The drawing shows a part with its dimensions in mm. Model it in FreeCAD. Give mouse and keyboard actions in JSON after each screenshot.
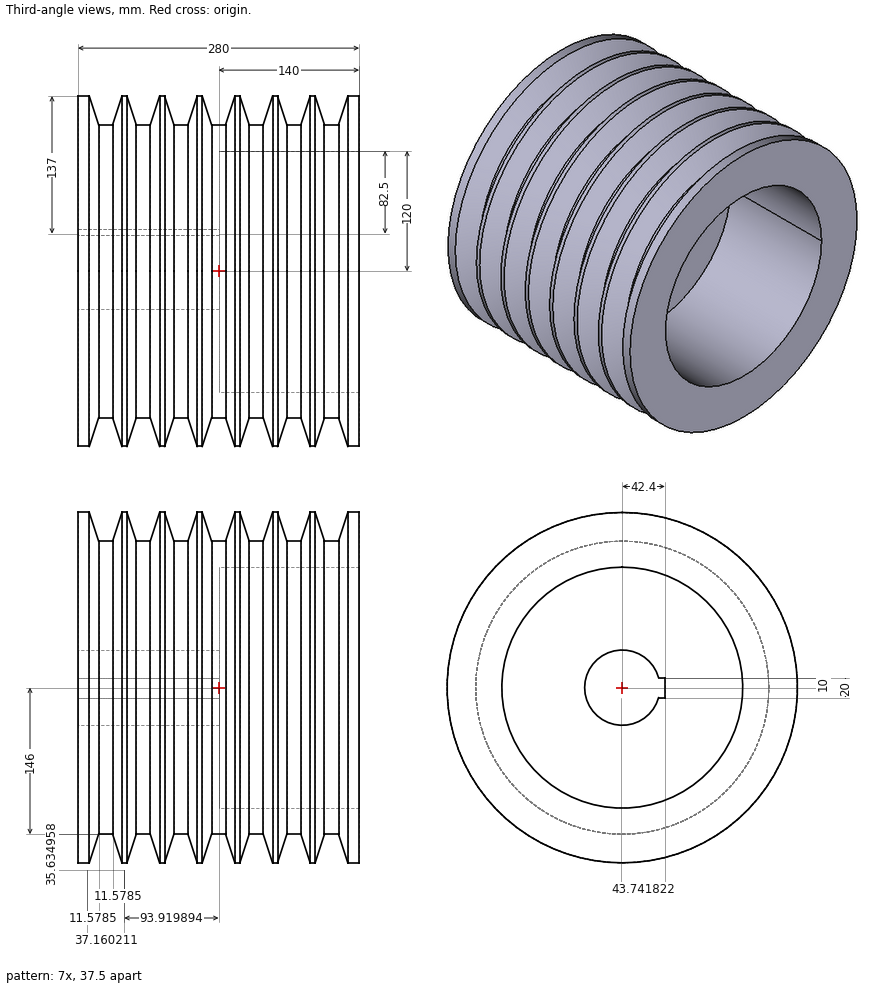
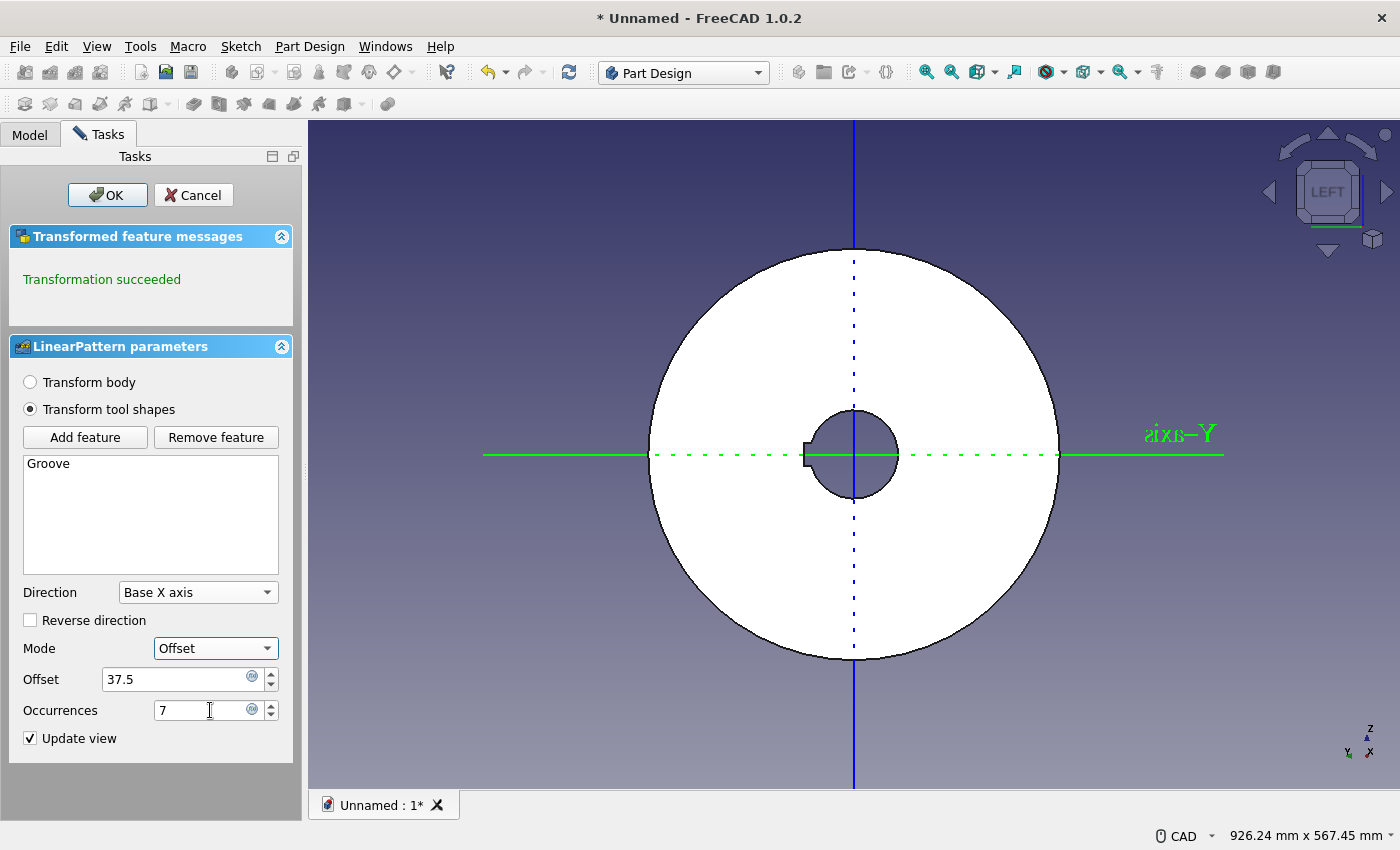
{"action": "left_click", "coordinate": [108, 195]}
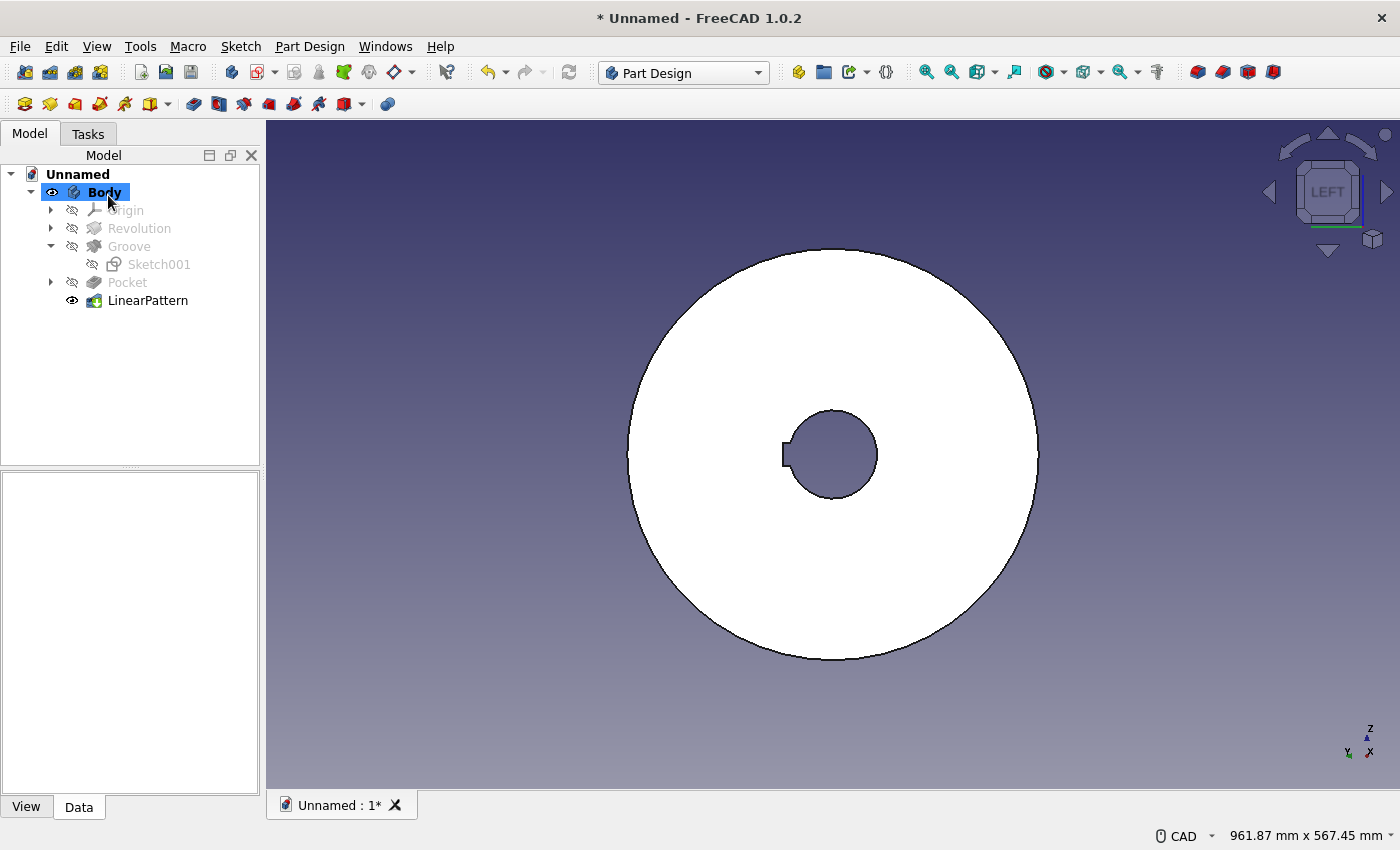
{"action": "key", "text": "0"}